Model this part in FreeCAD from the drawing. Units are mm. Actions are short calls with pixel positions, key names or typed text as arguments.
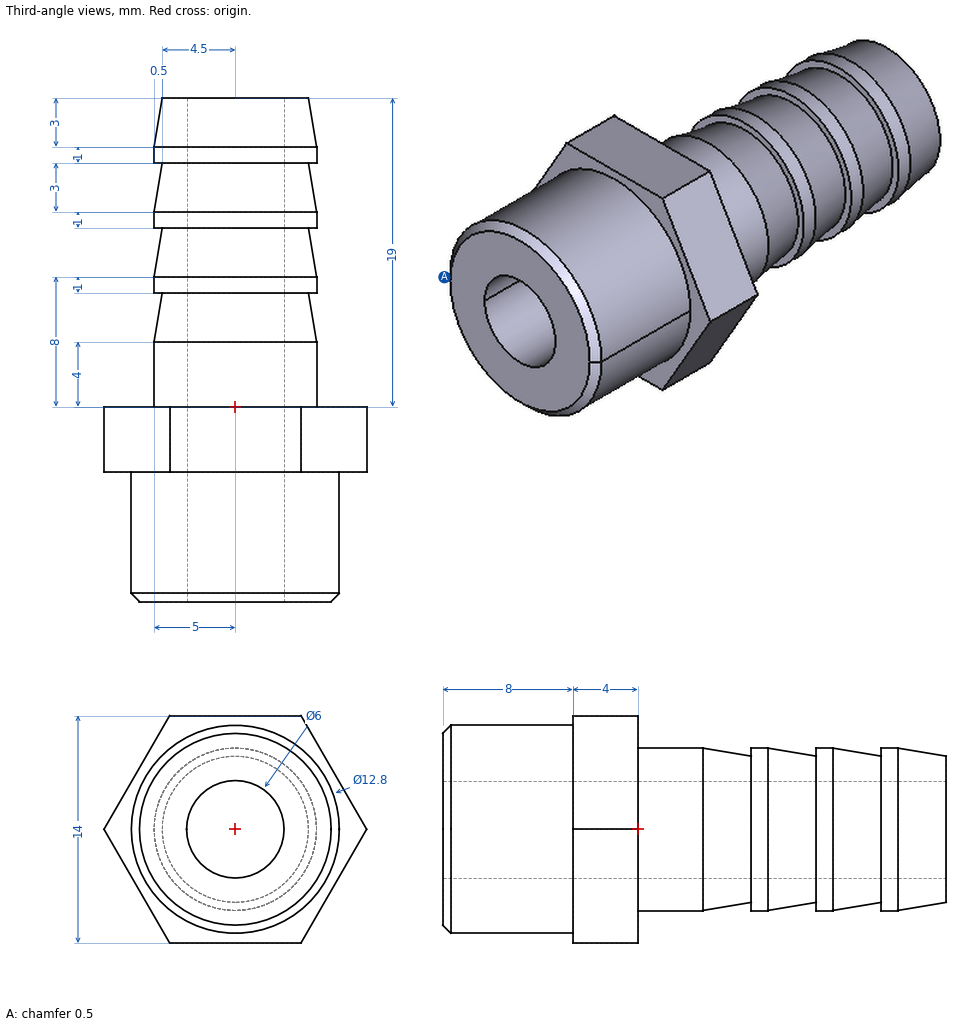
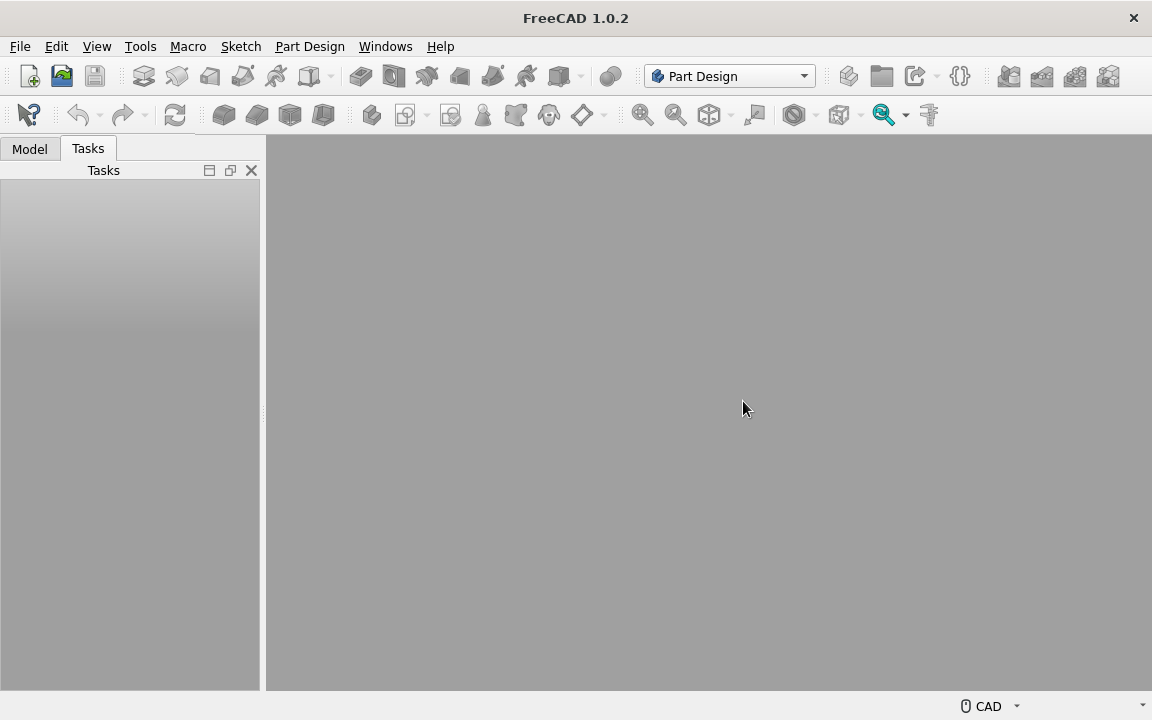
click(29, 76)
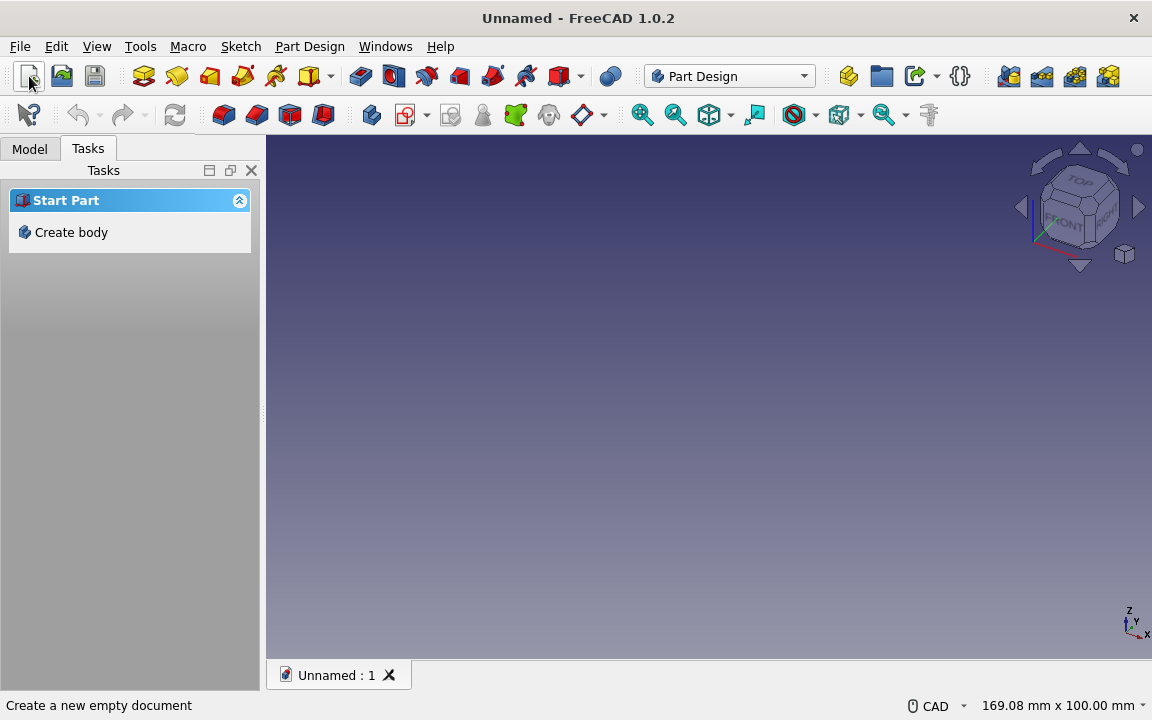
click(404, 116)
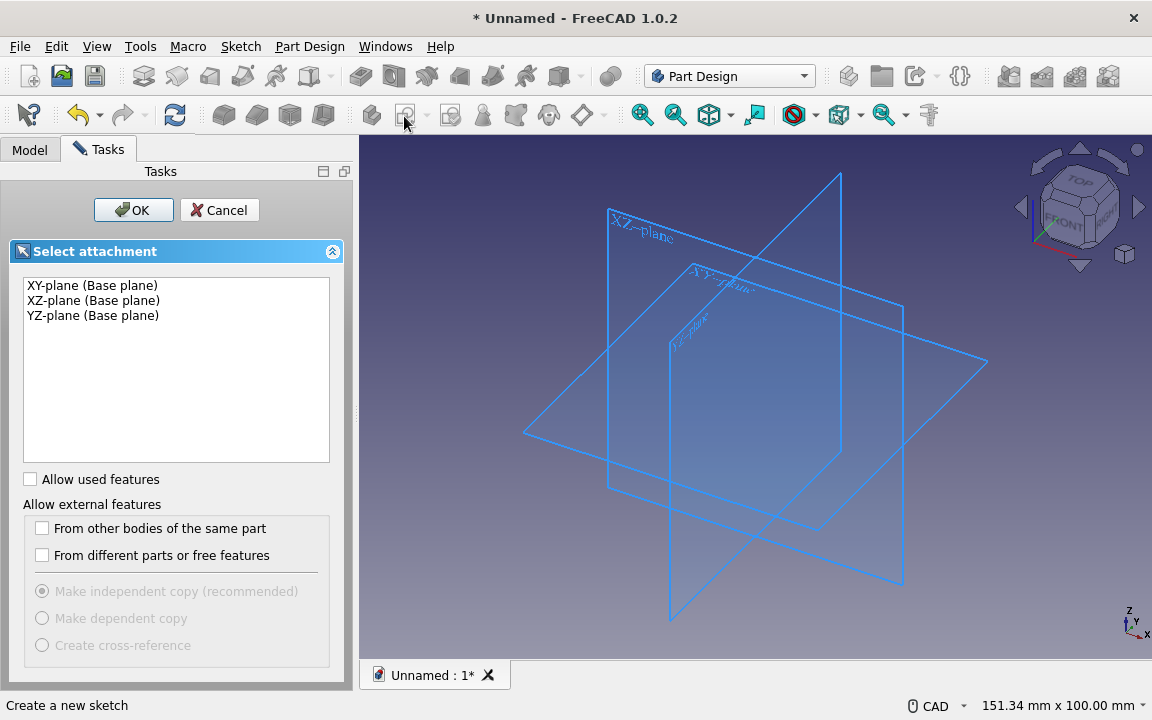
click(84, 286)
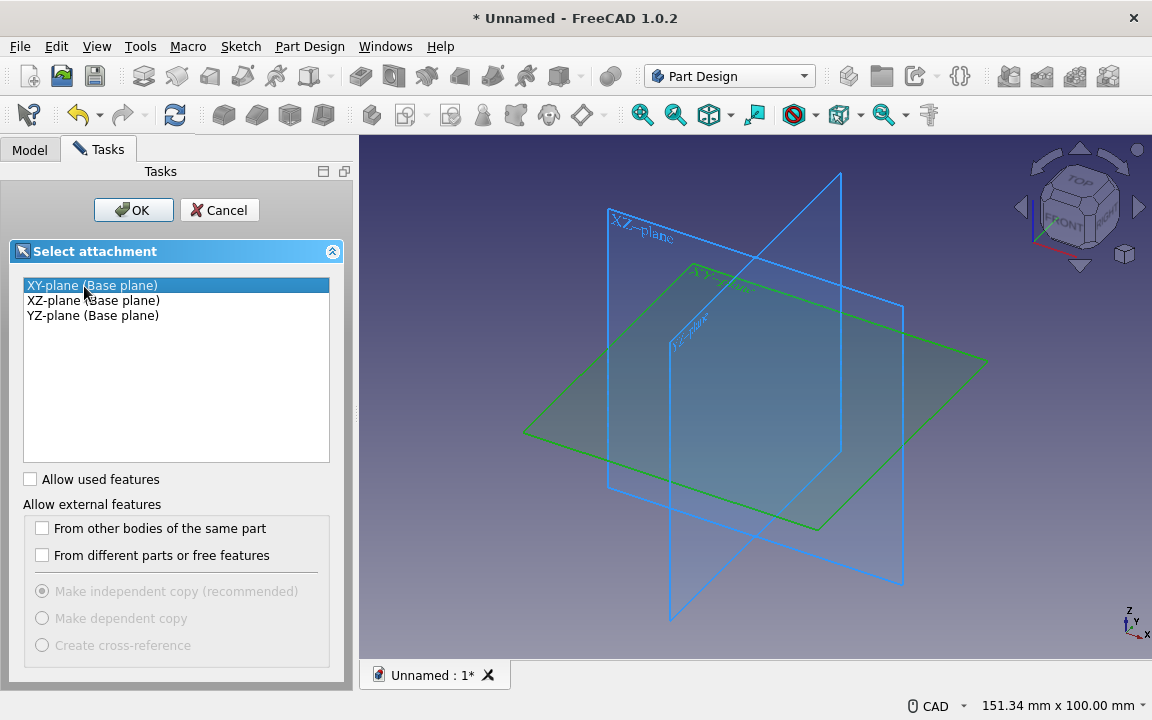
click(134, 210)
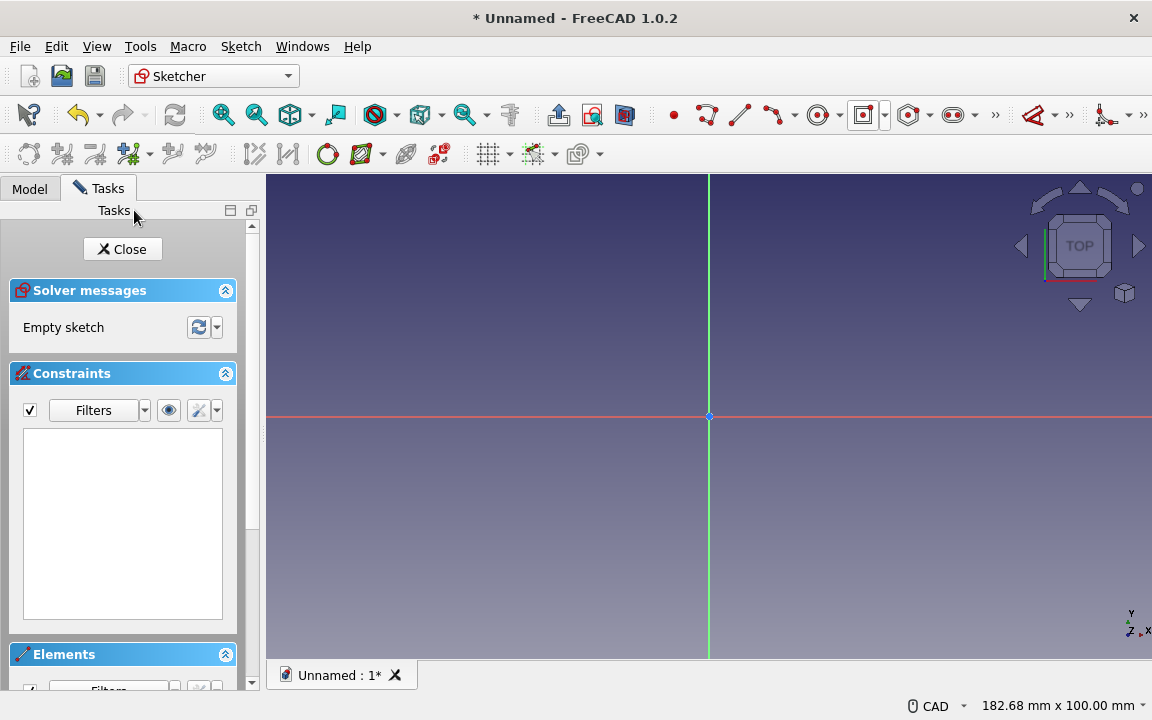
scroll(721, 351, up, 6)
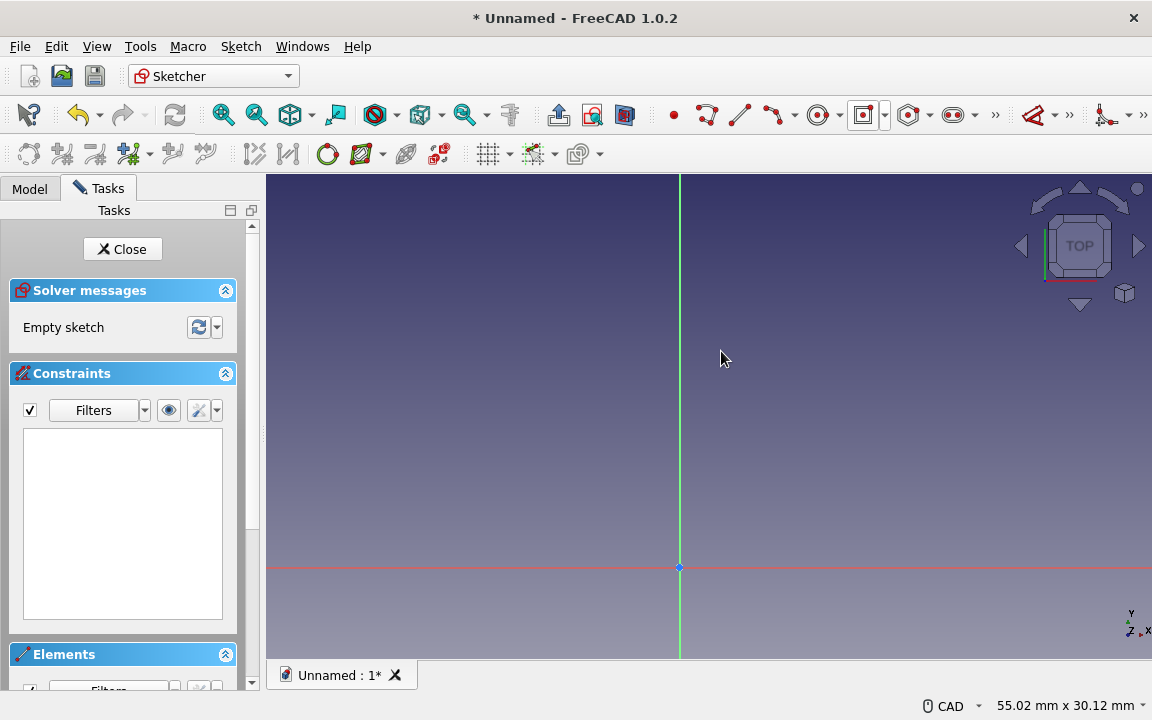
click(707, 116)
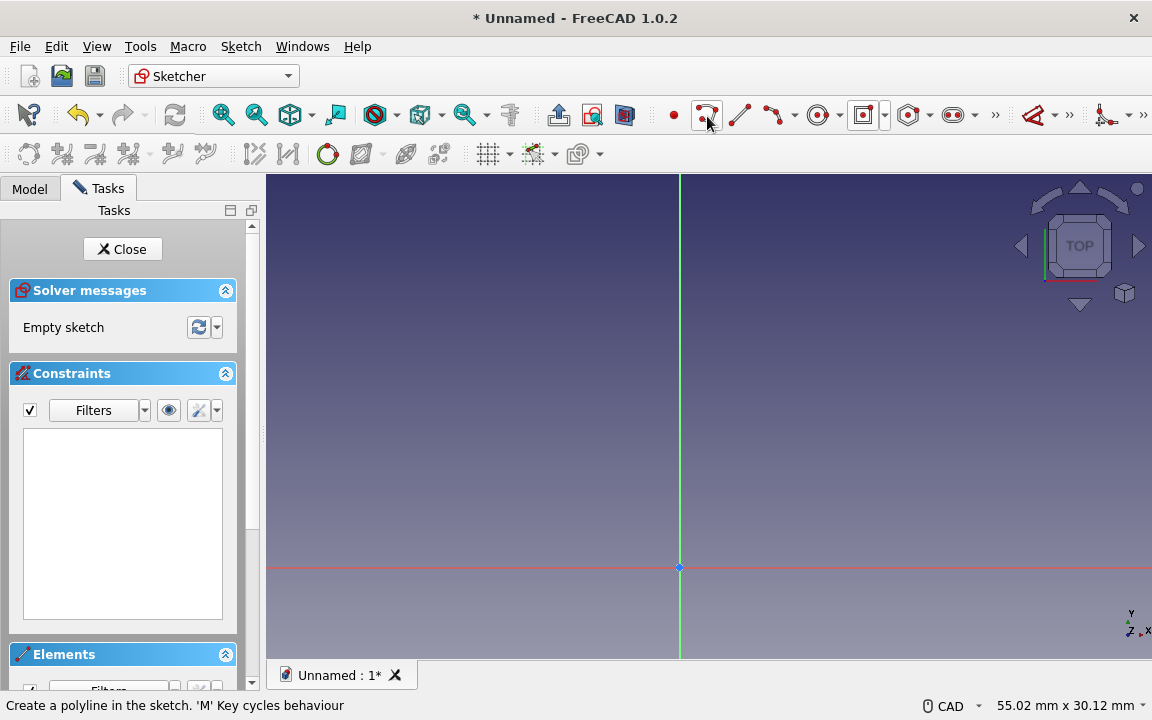
click(680, 568)
click(671, 262)
click(608, 262)
click(599, 310)
click(599, 326)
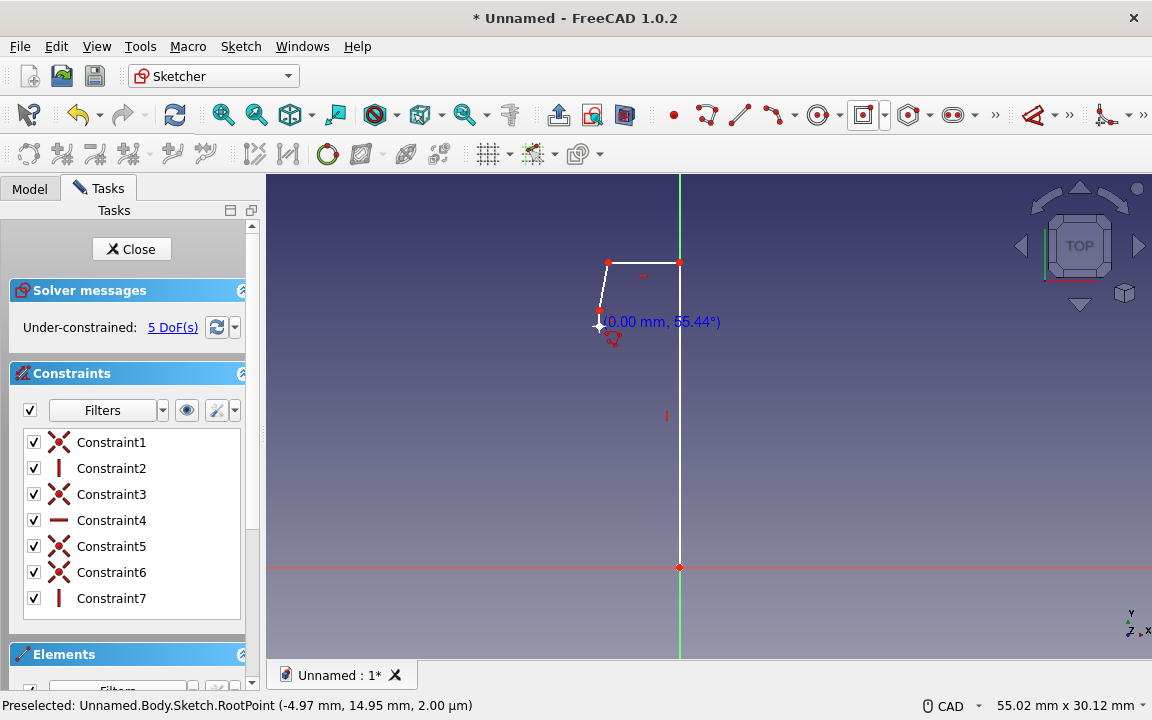
scroll(608, 326, up, 4)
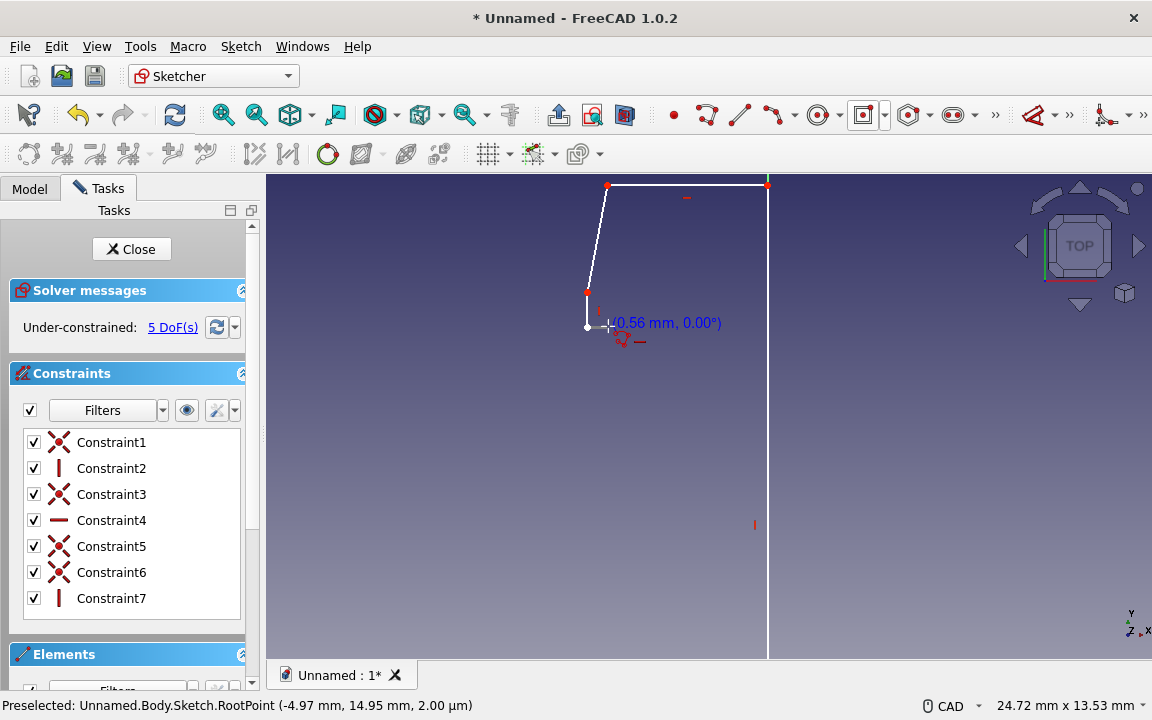
click(606, 326)
click(589, 433)
click(589, 469)
click(606, 469)
click(589, 577)
click(589, 612)
click(606, 612)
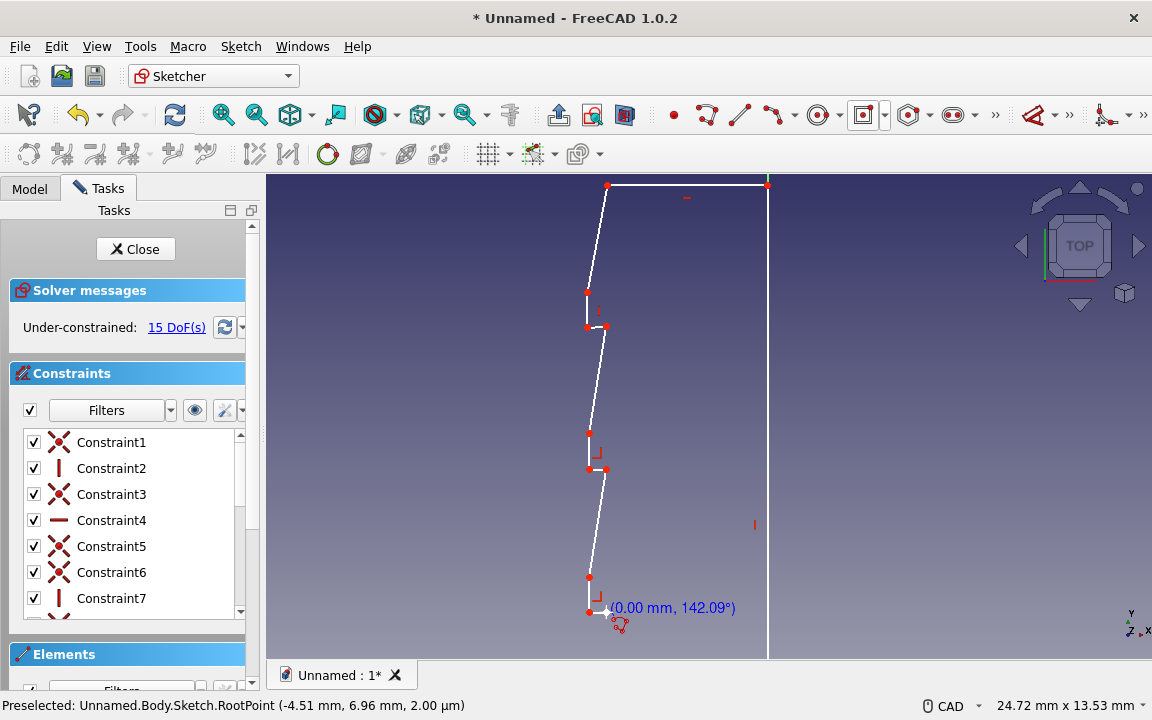
scroll(610, 330, down, 4)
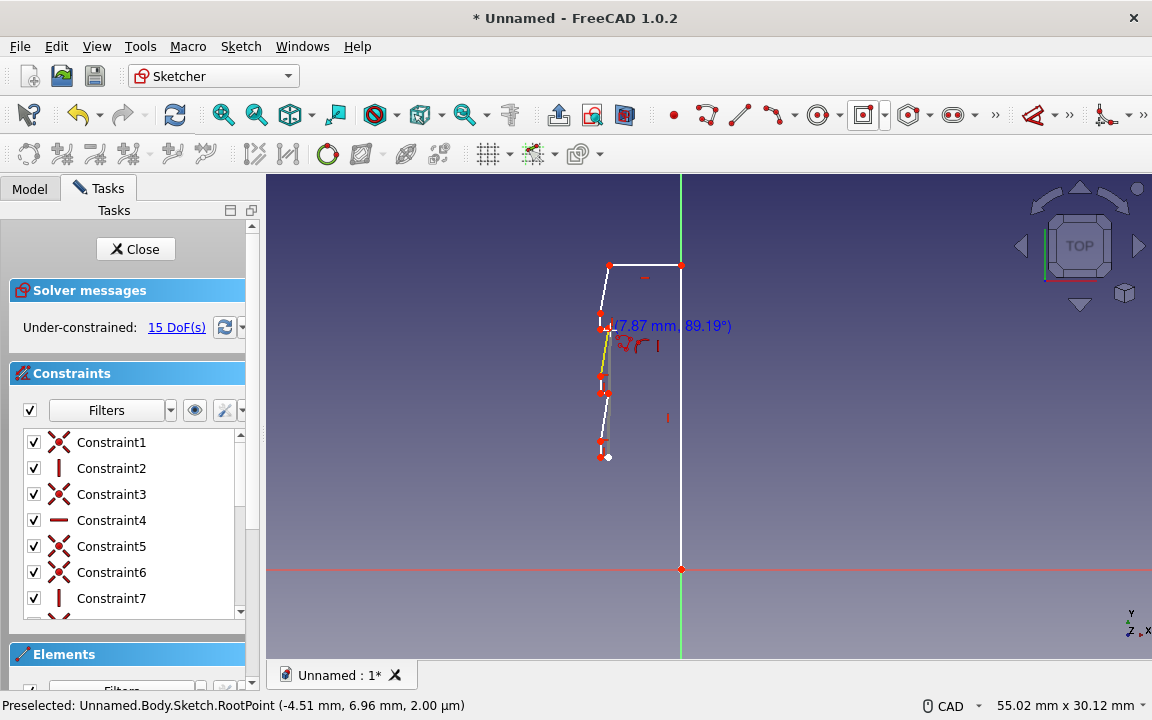
click(601, 505)
click(601, 561)
click(681, 570)
key(Escape)
key(Escape)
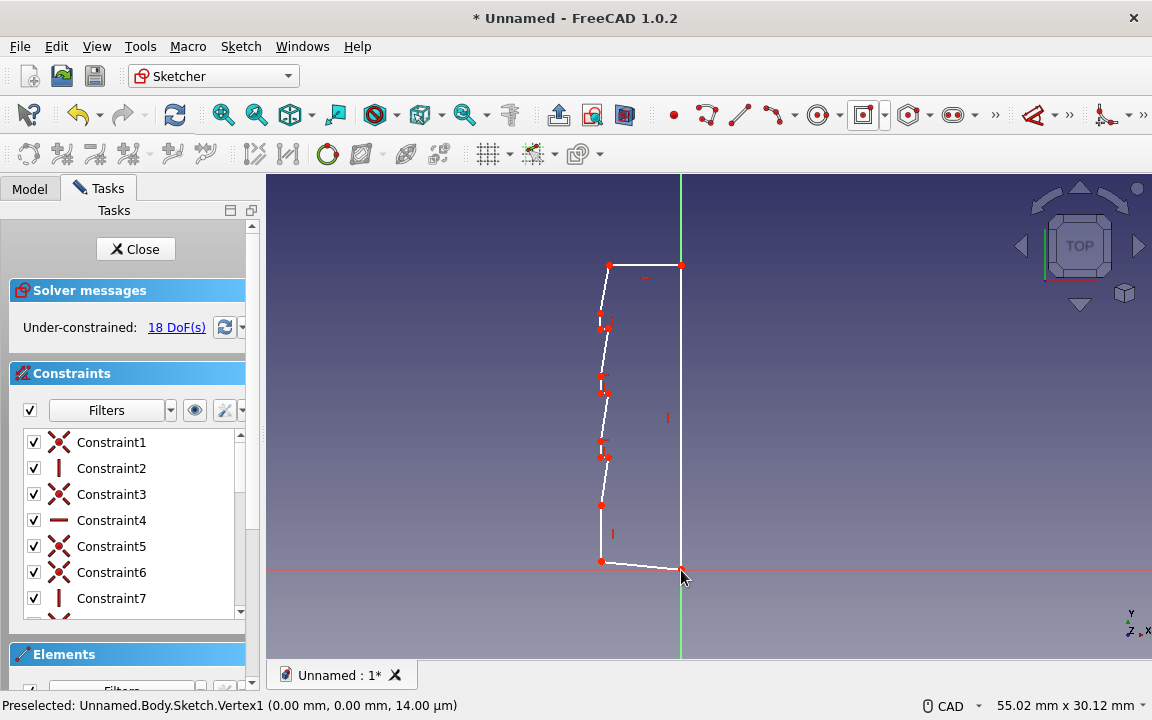
scroll(604, 329, up, 7)